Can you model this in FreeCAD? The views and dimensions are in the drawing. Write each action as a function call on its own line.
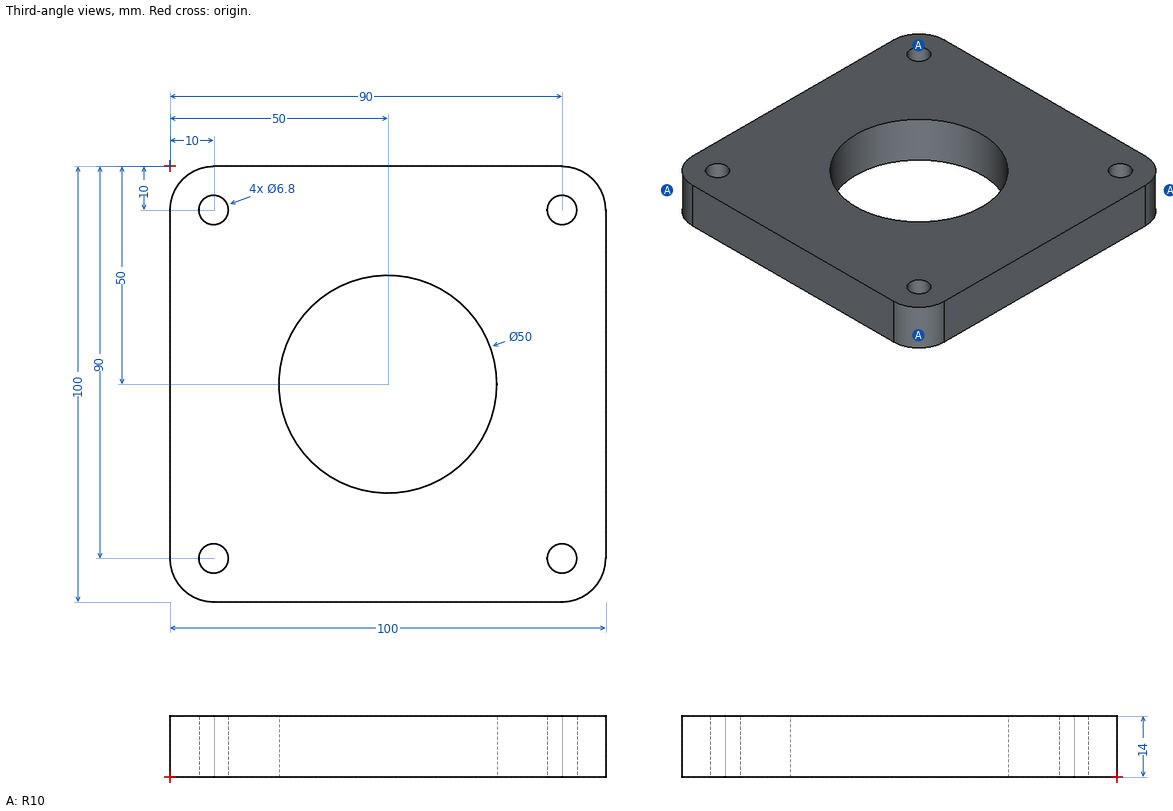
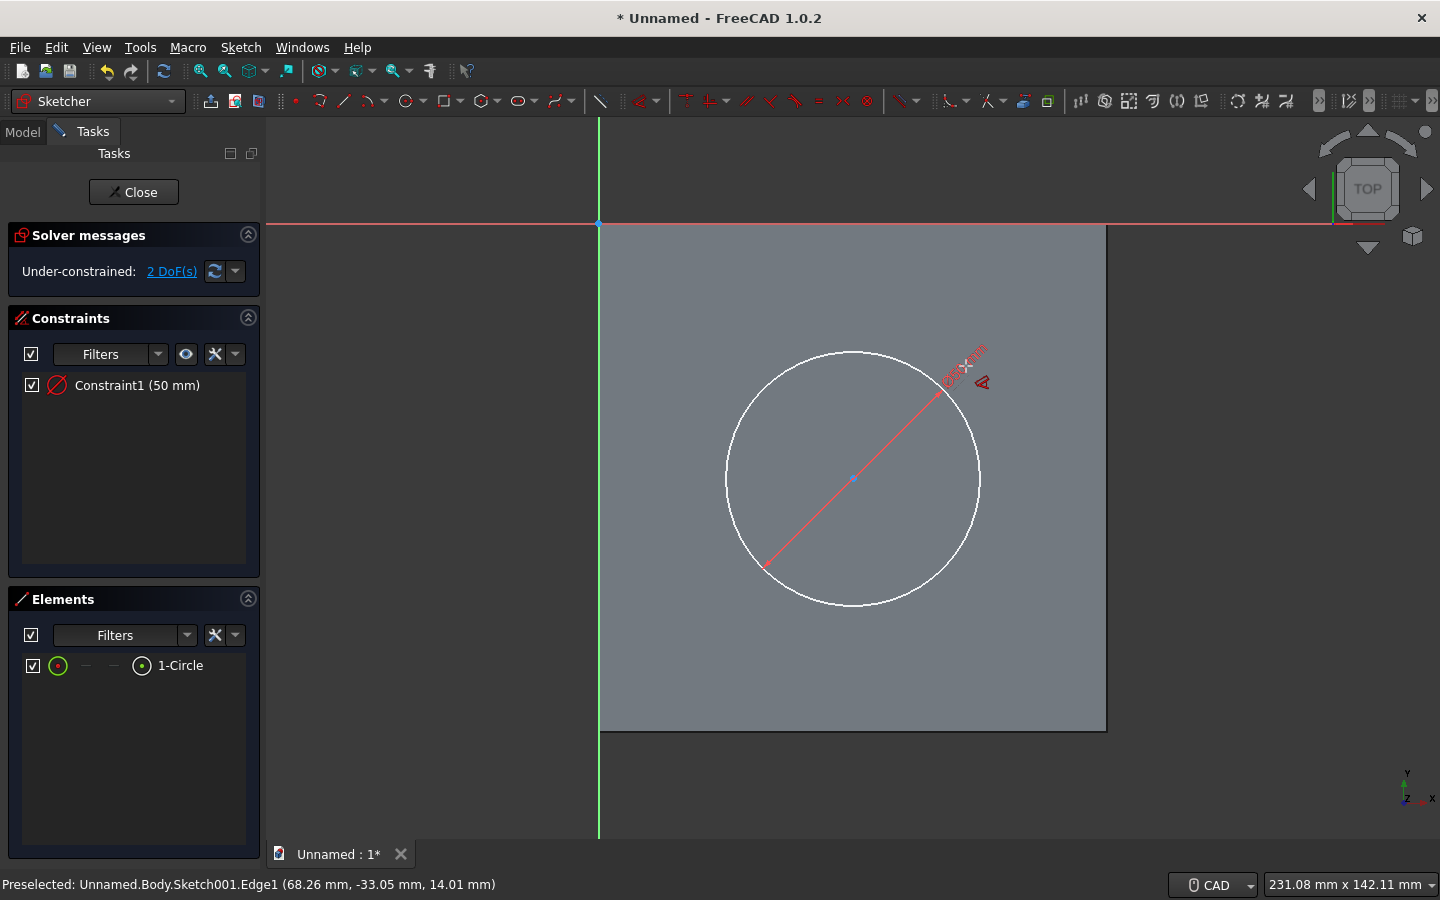
click(853, 479)
click(726, 190)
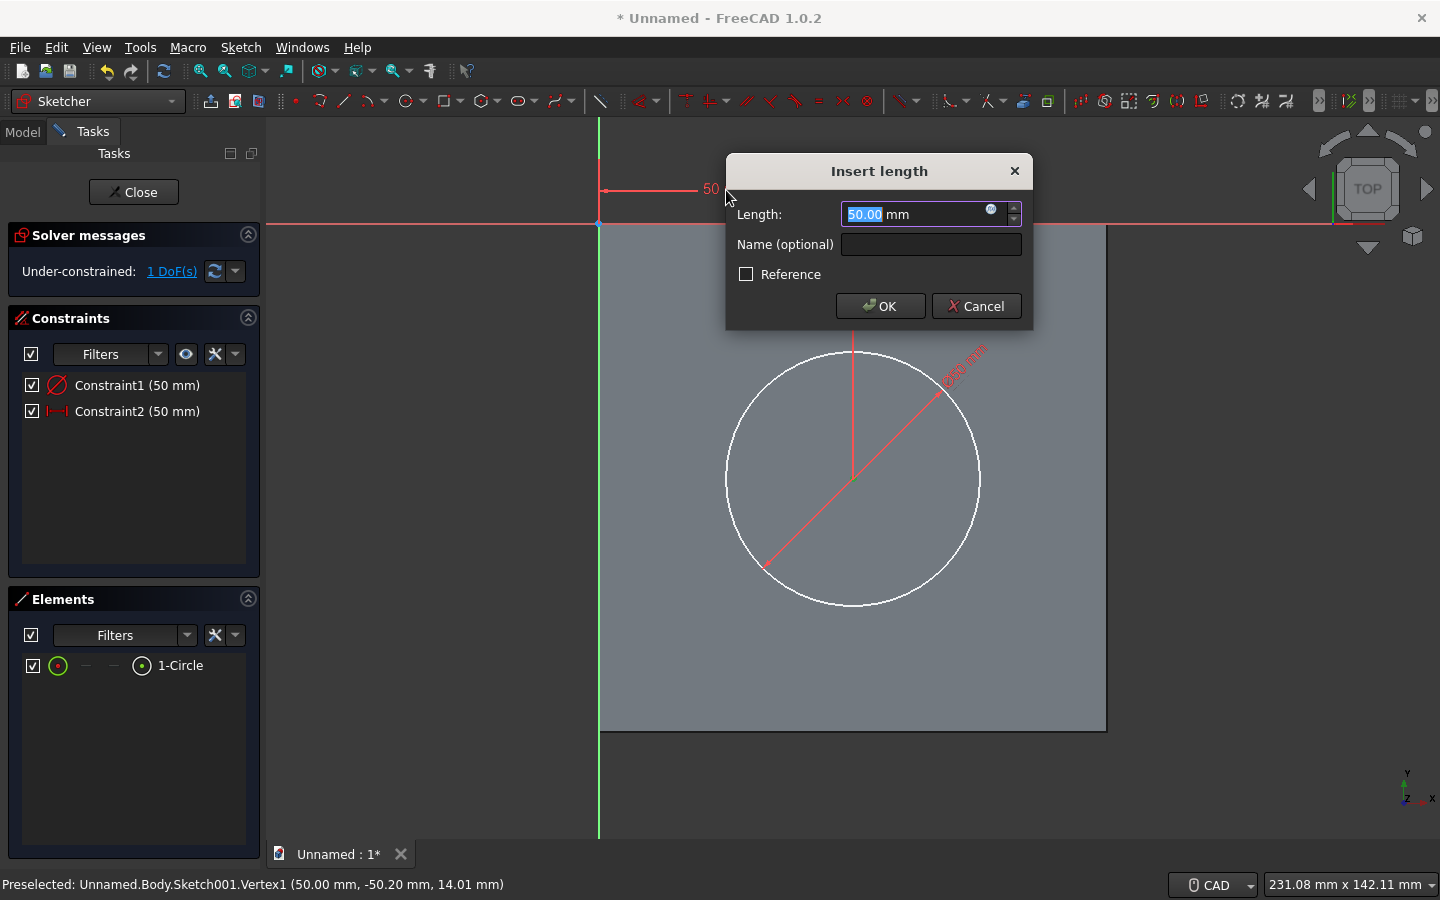
text(50)
key(Return)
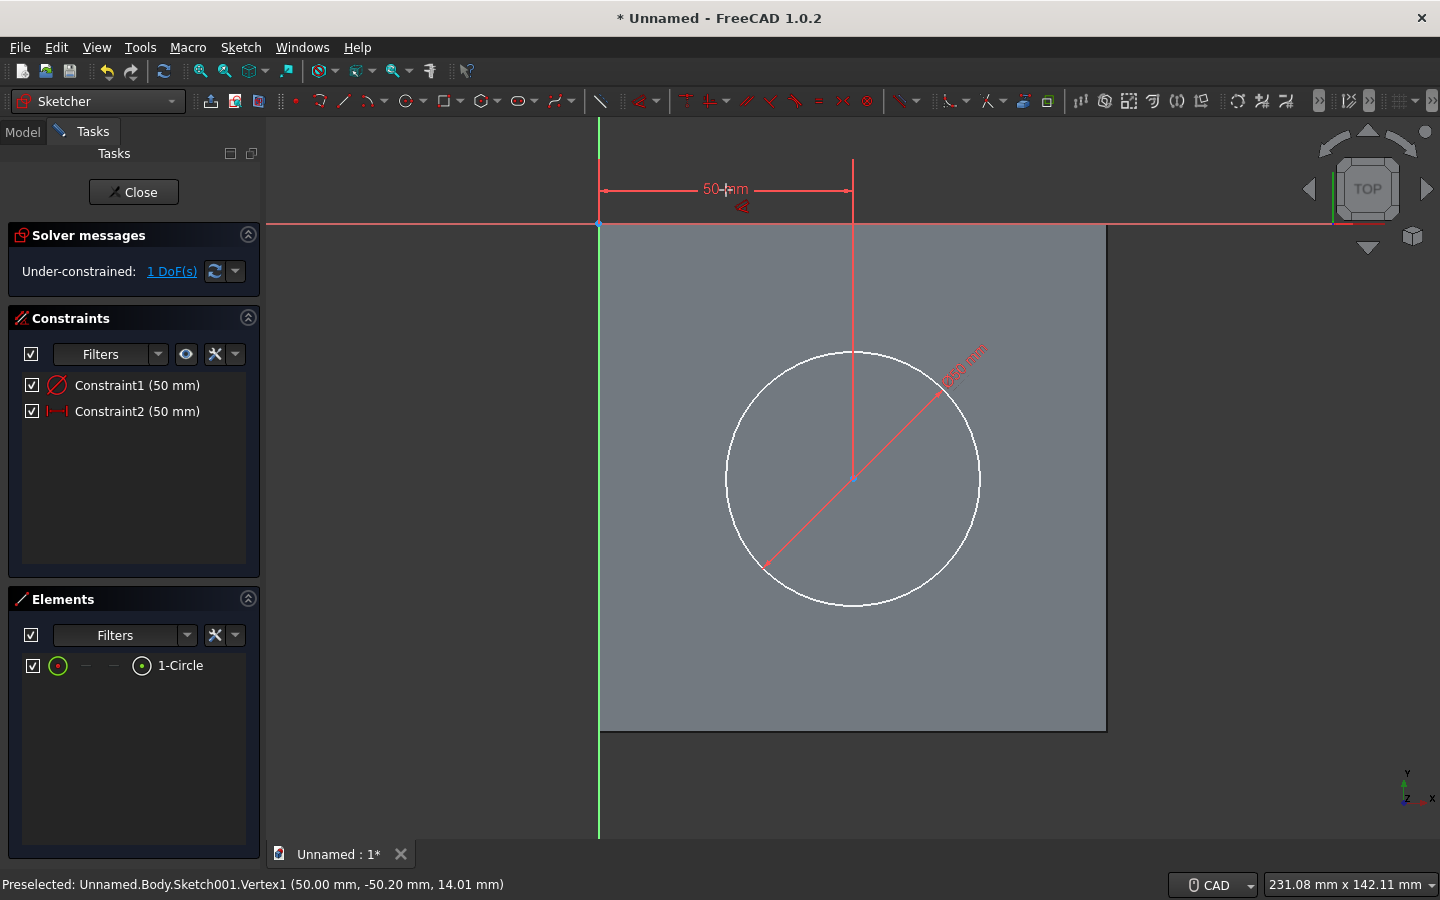
click(853, 479)
click(565, 351)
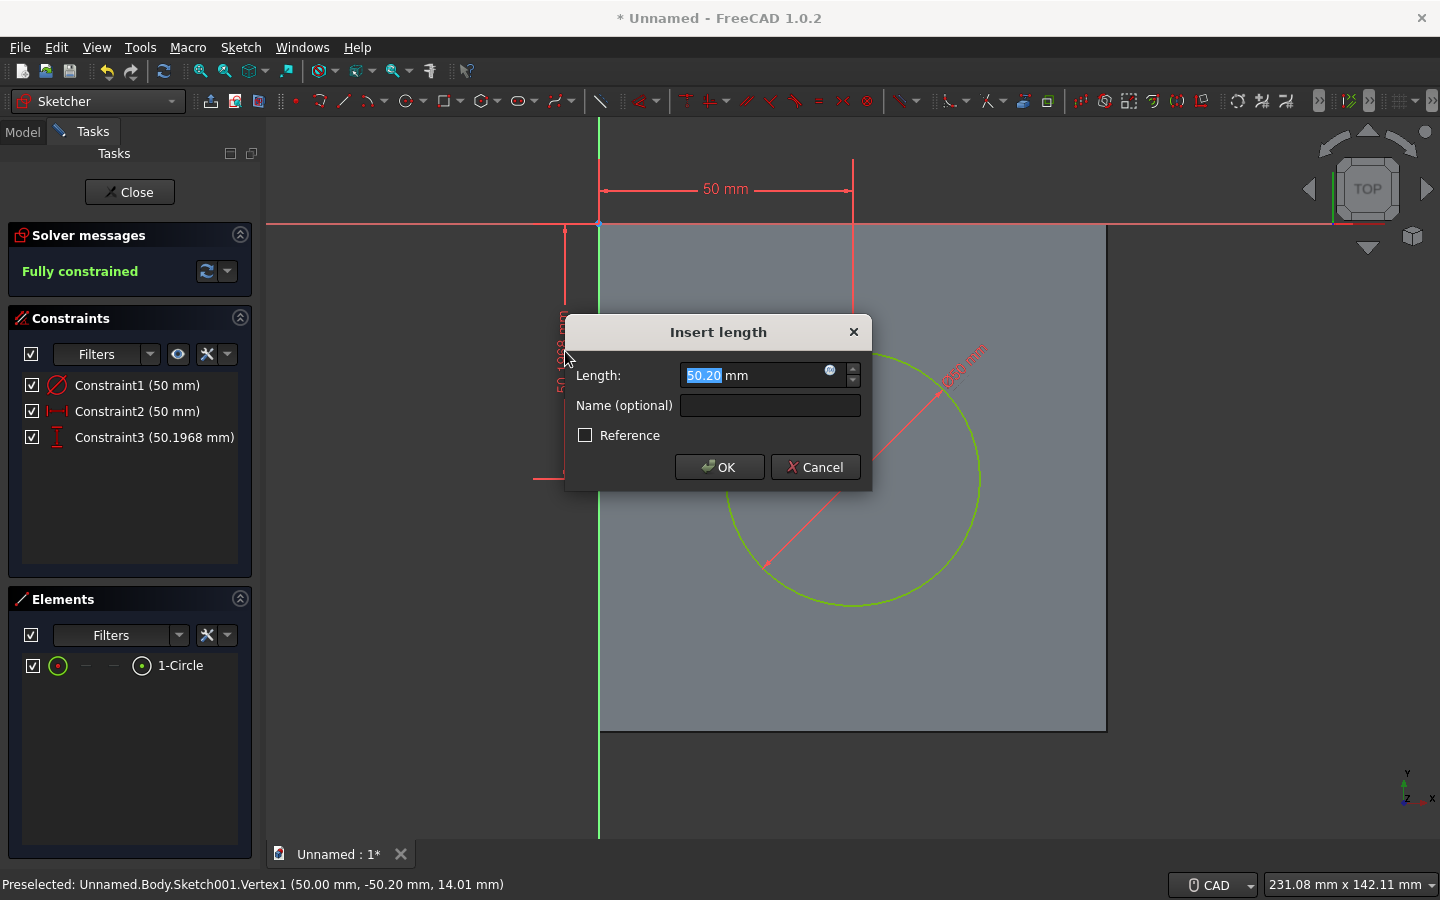
text(50)
key(Return)
key(Escape)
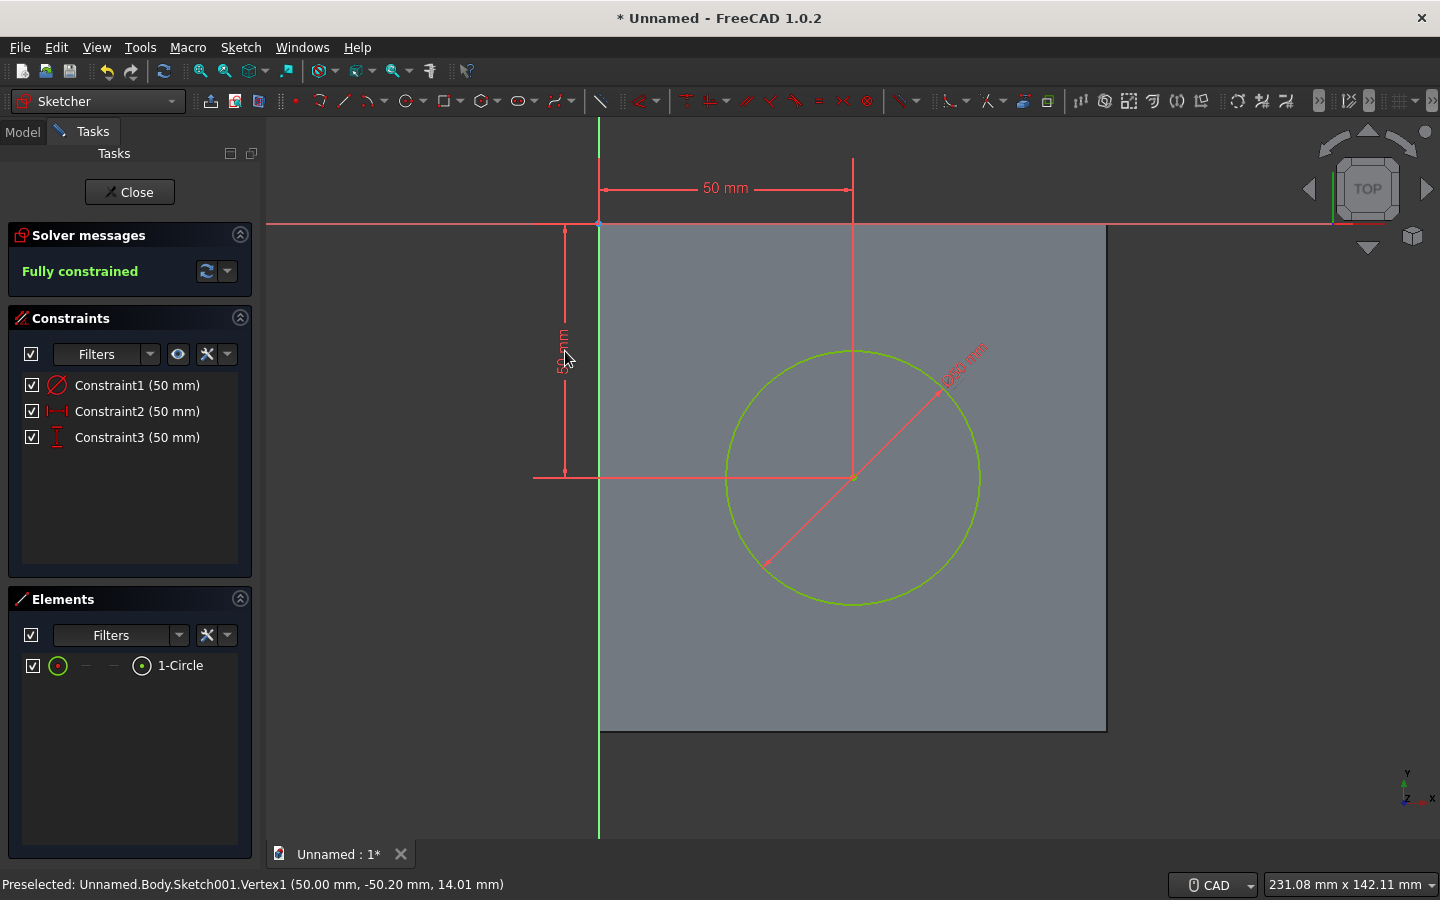
click(130, 192)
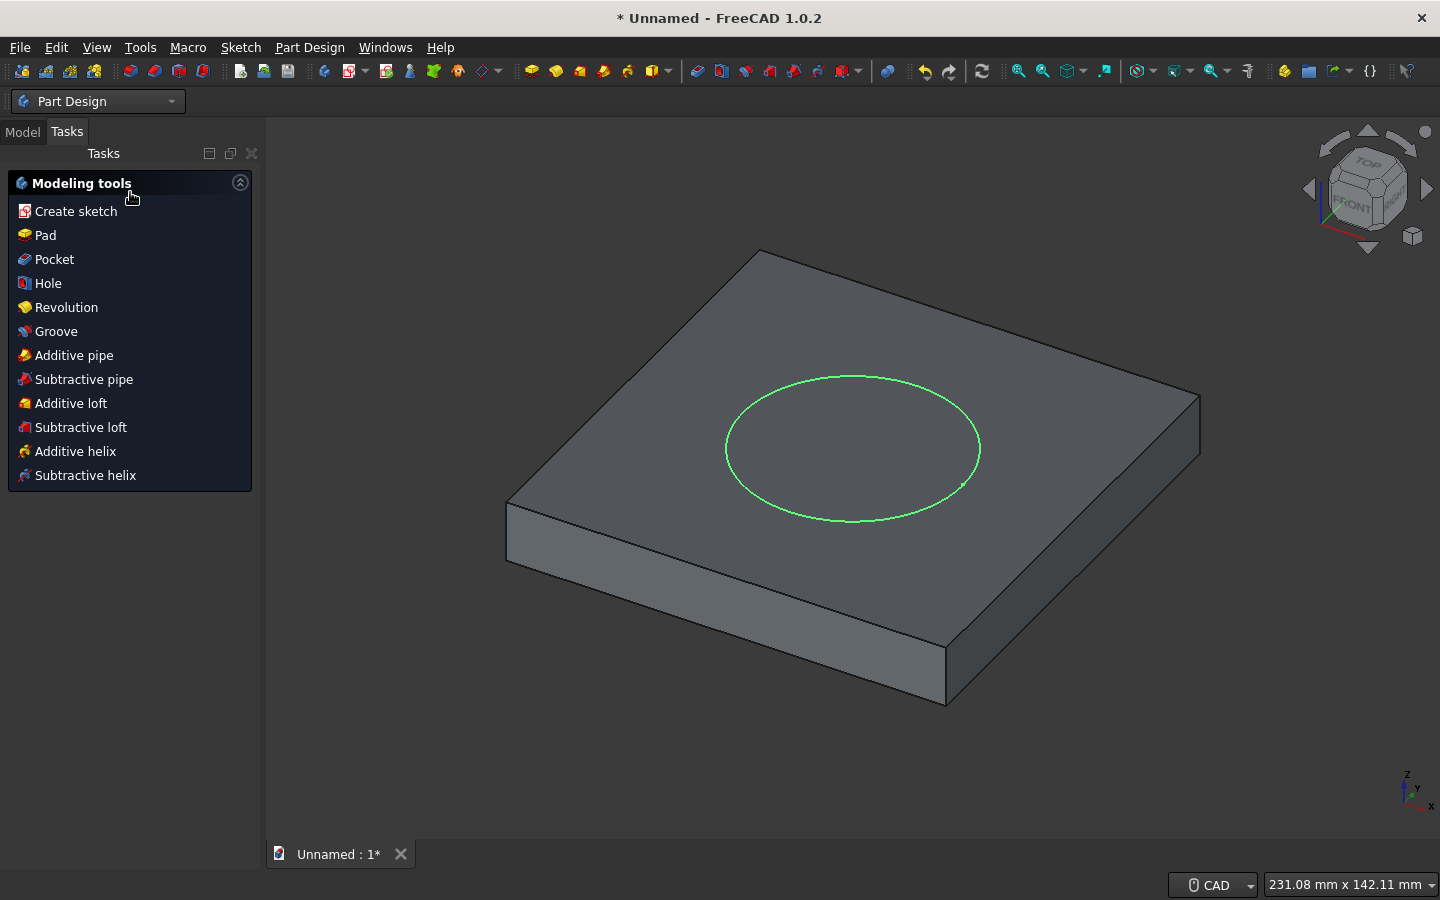
click(698, 72)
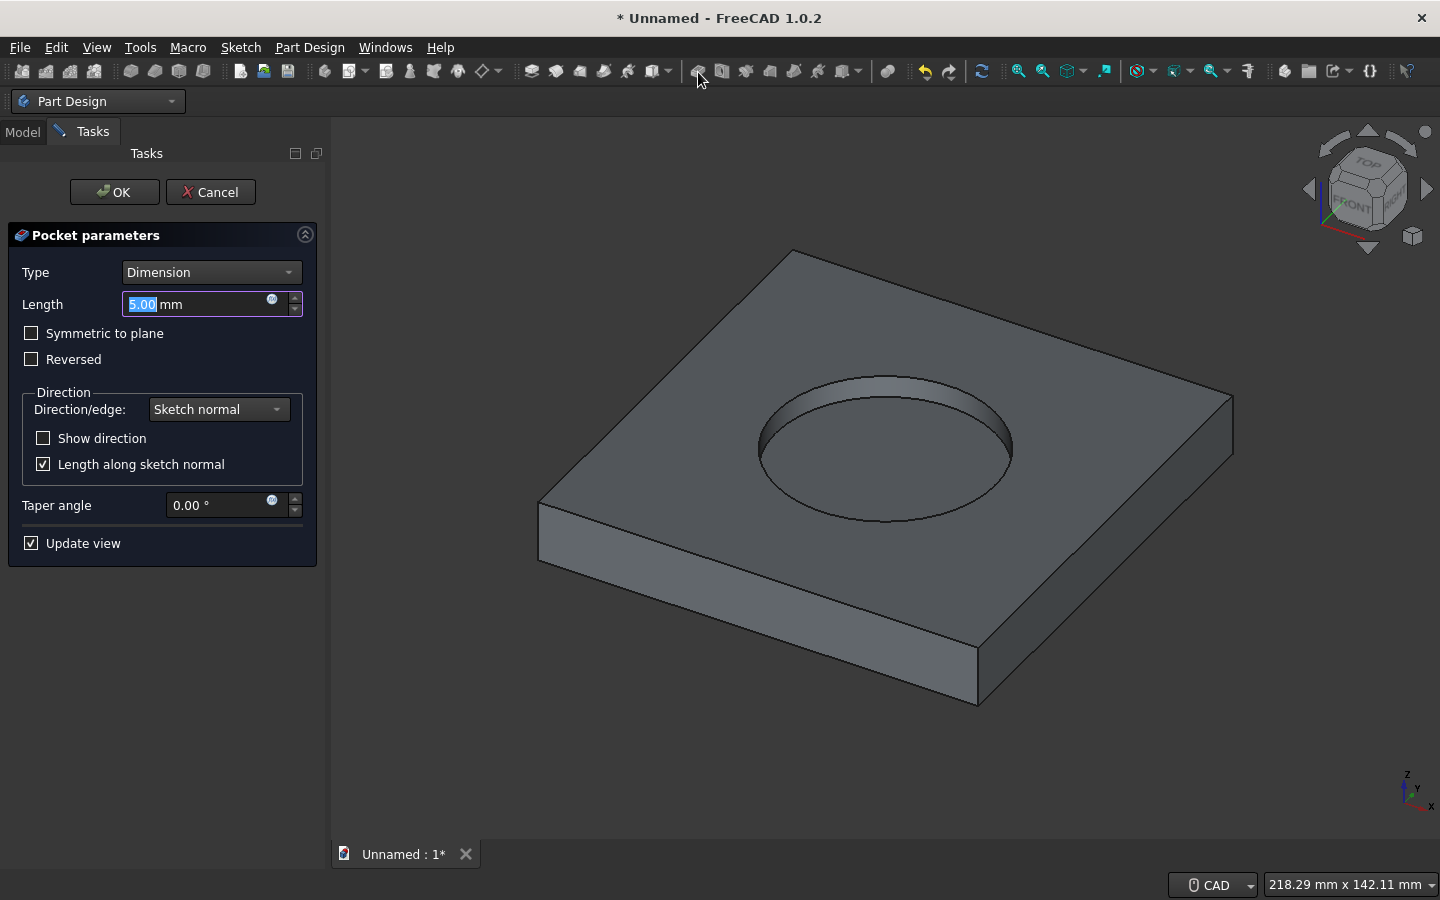
click(212, 272)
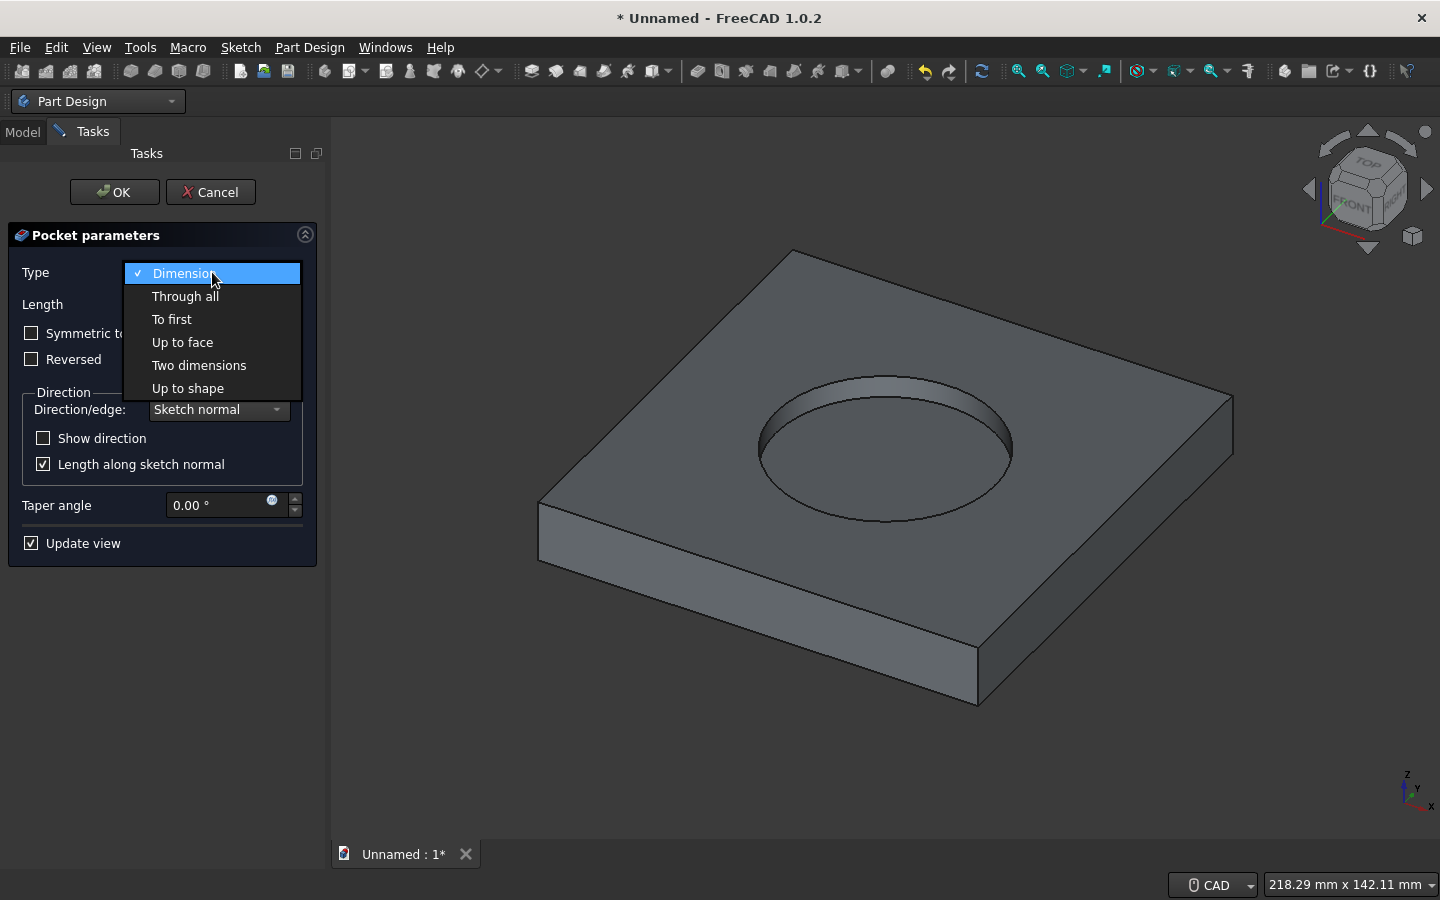
click(212, 296)